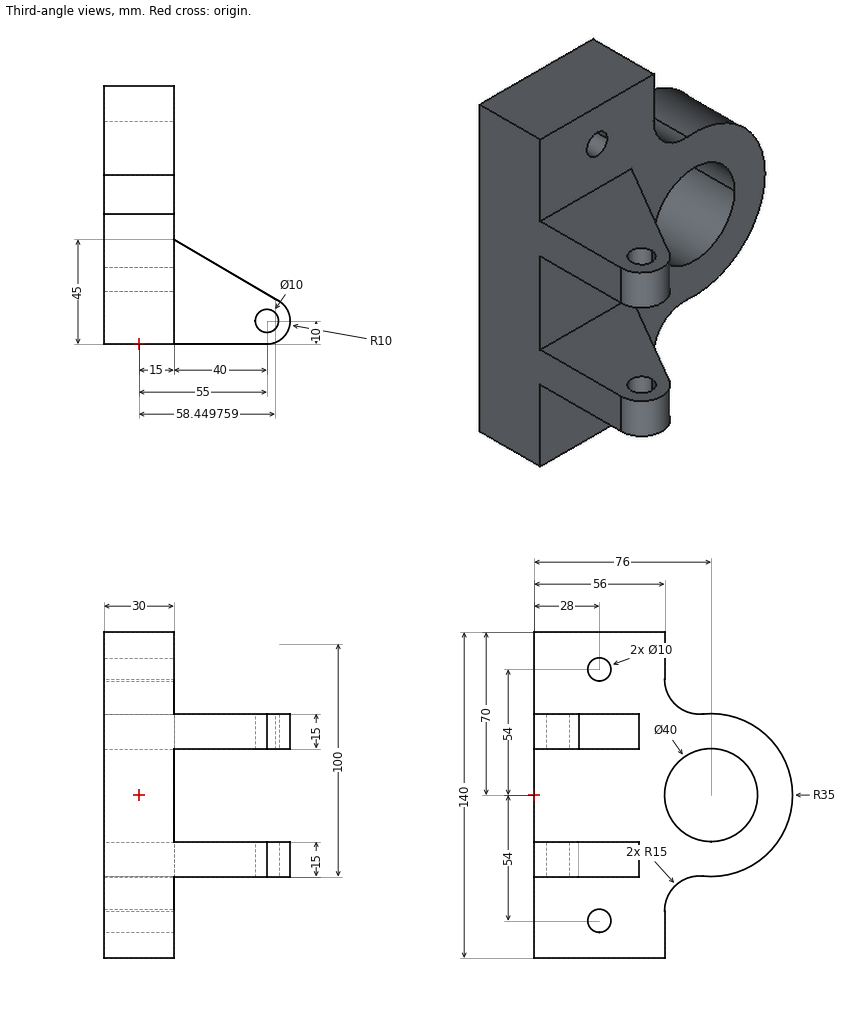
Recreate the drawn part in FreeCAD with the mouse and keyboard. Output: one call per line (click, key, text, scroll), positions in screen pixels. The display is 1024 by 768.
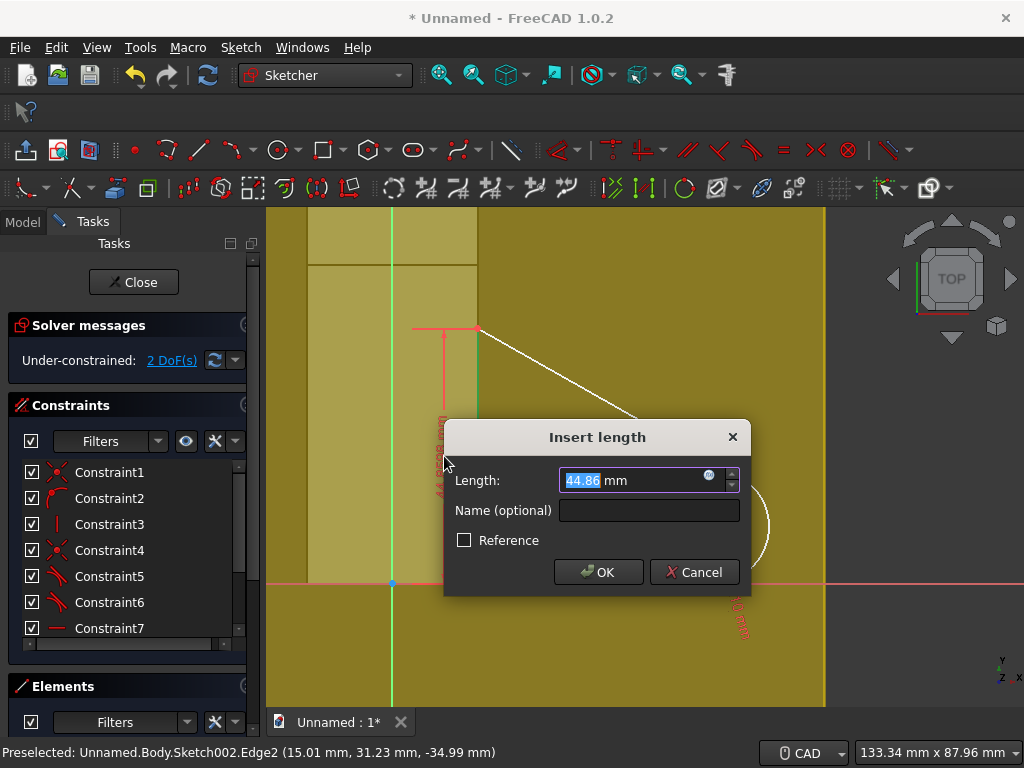
text(45)
key(Return)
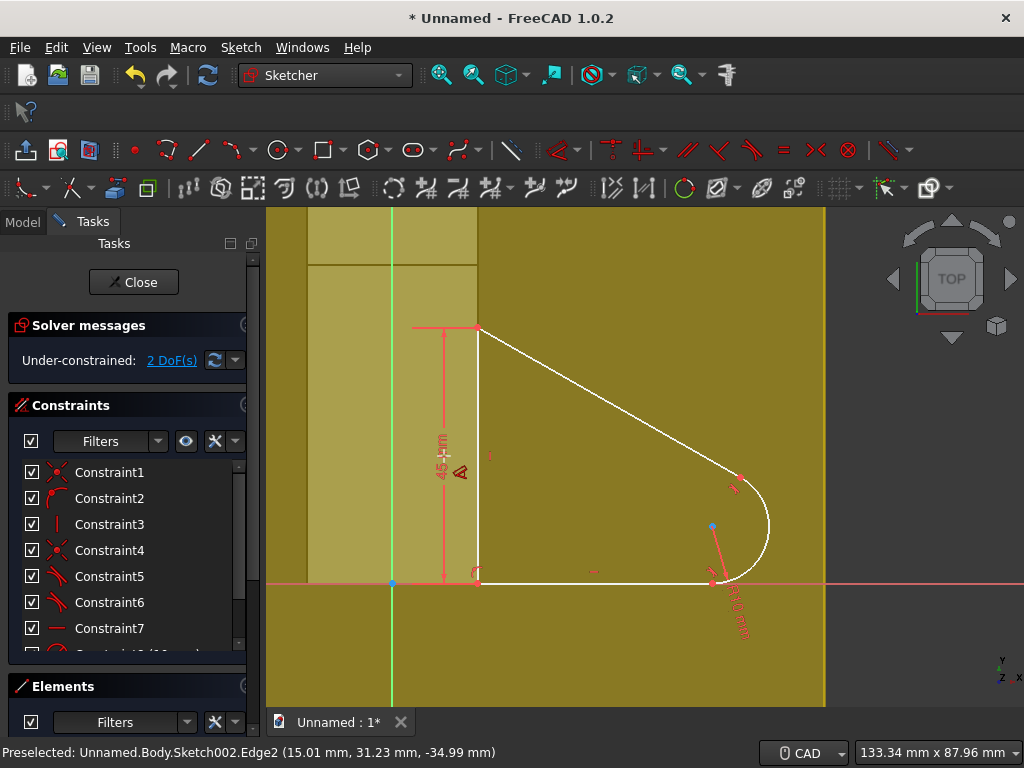
click(548, 584)
click(595, 618)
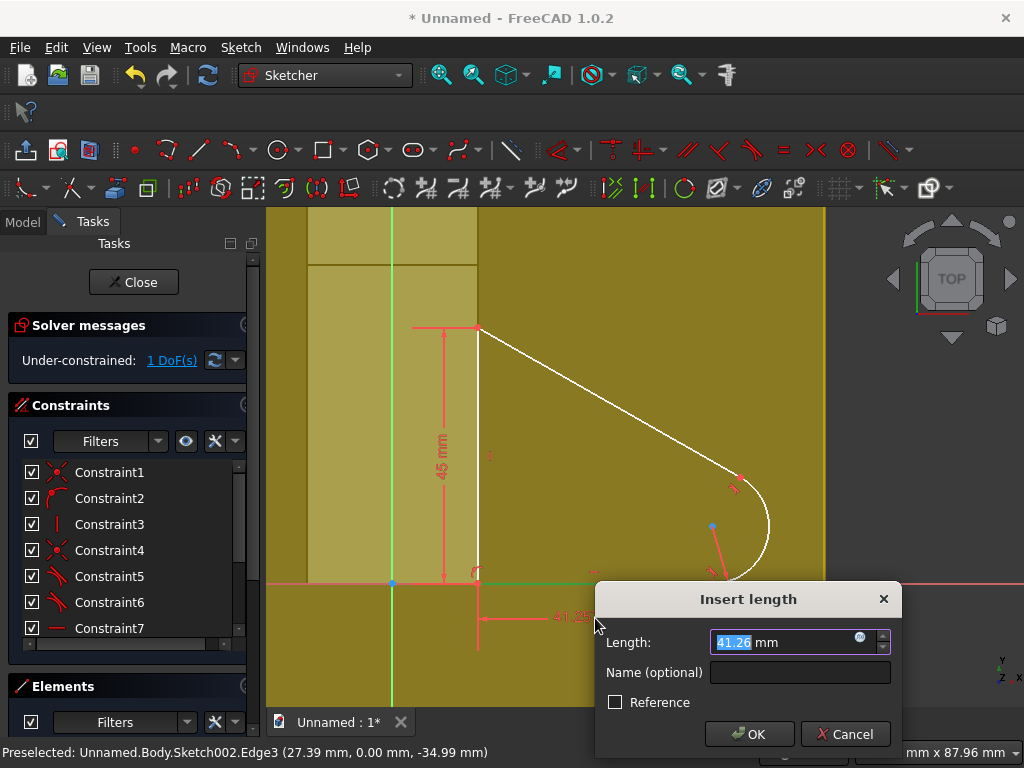
text(40)
key(Return)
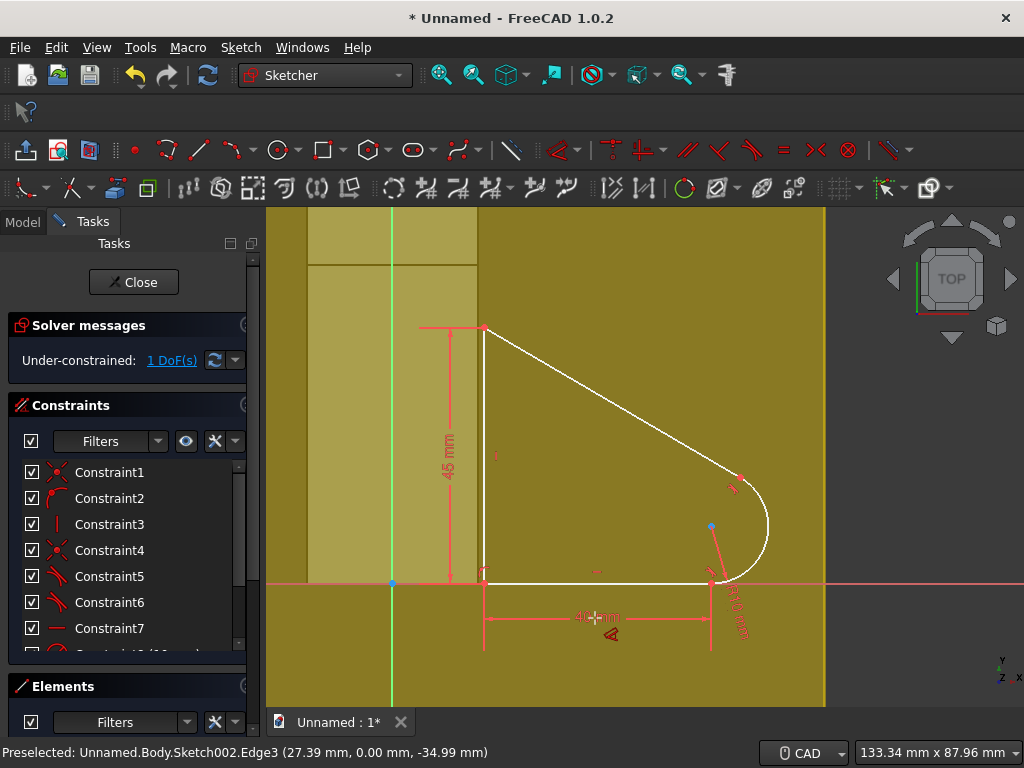
click(484, 328)
click(438, 618)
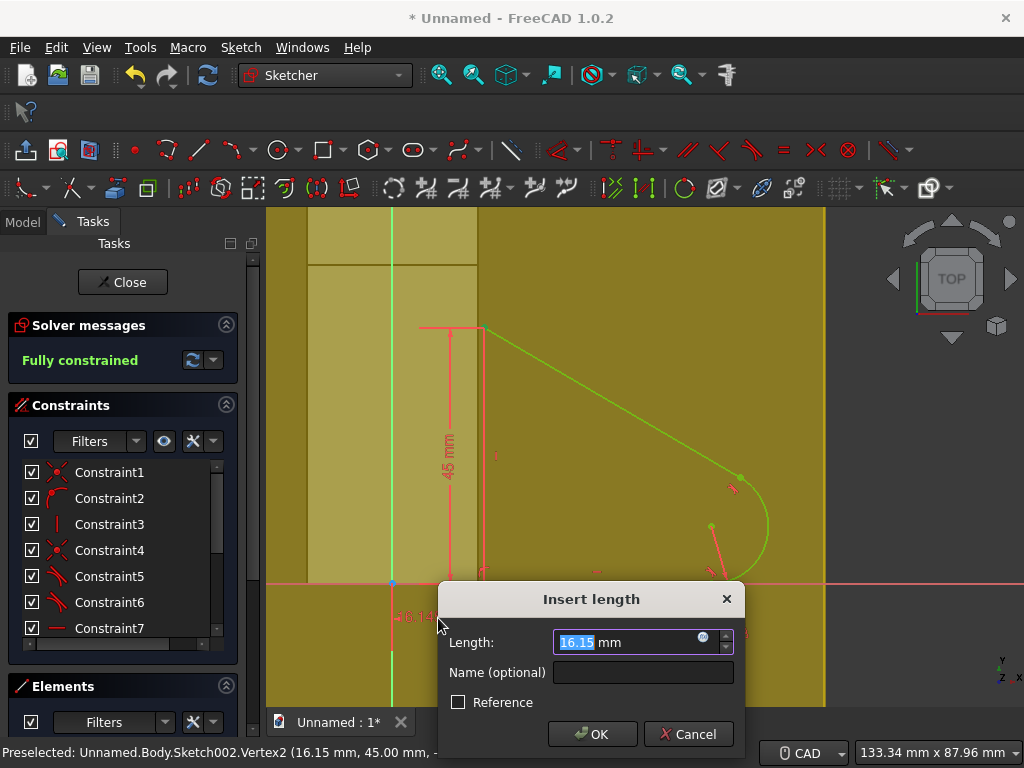
text(15)
key(Return)
key(Escape)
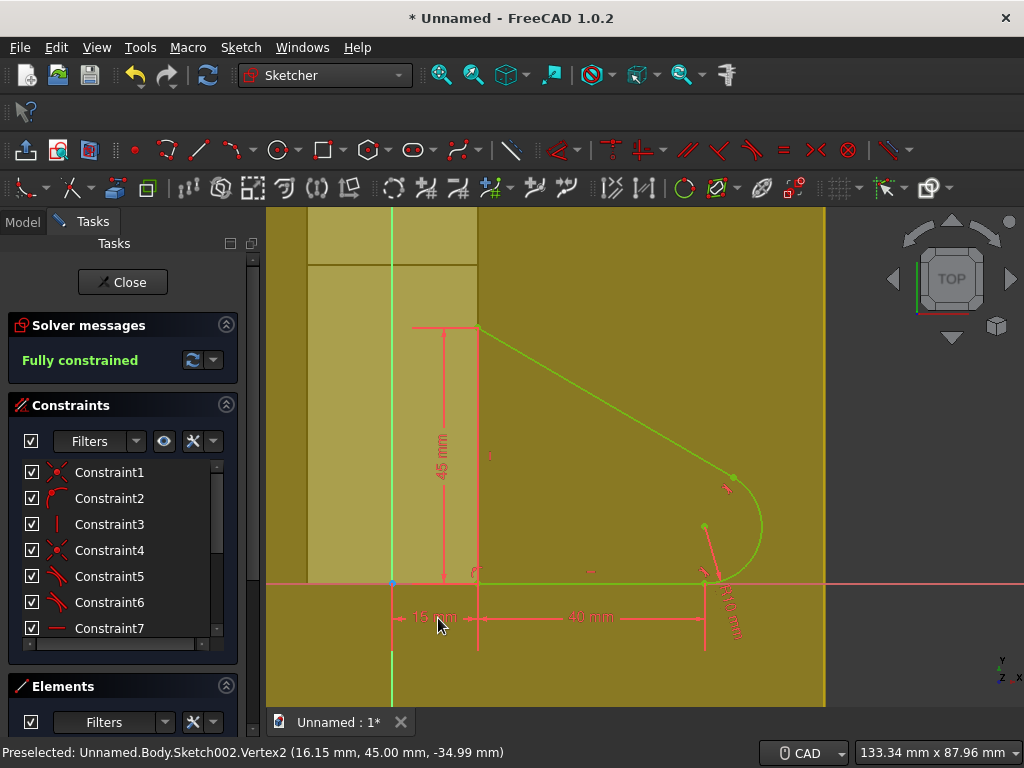
click(123, 282)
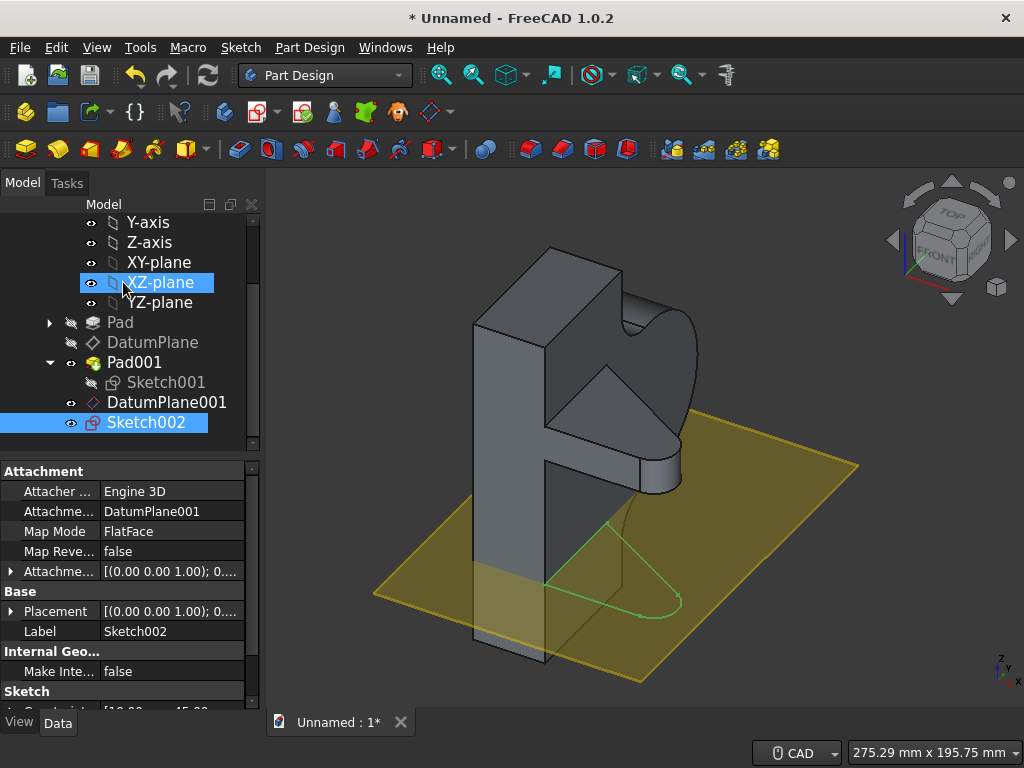
click(26, 150)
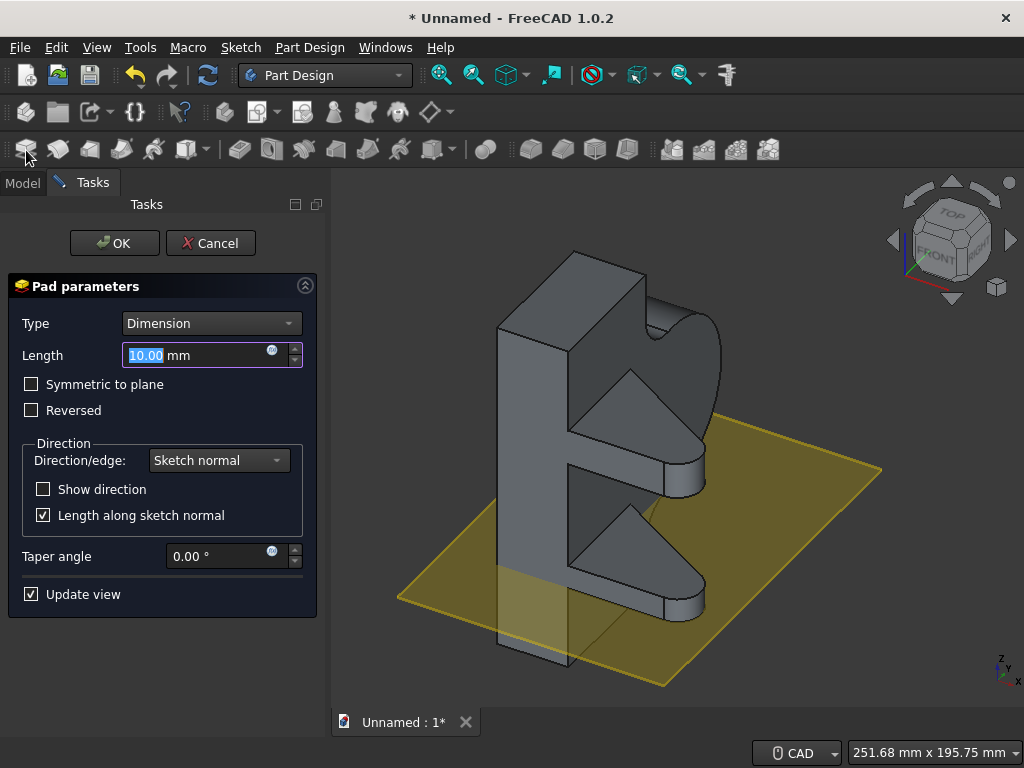
text(15)
key(Tab)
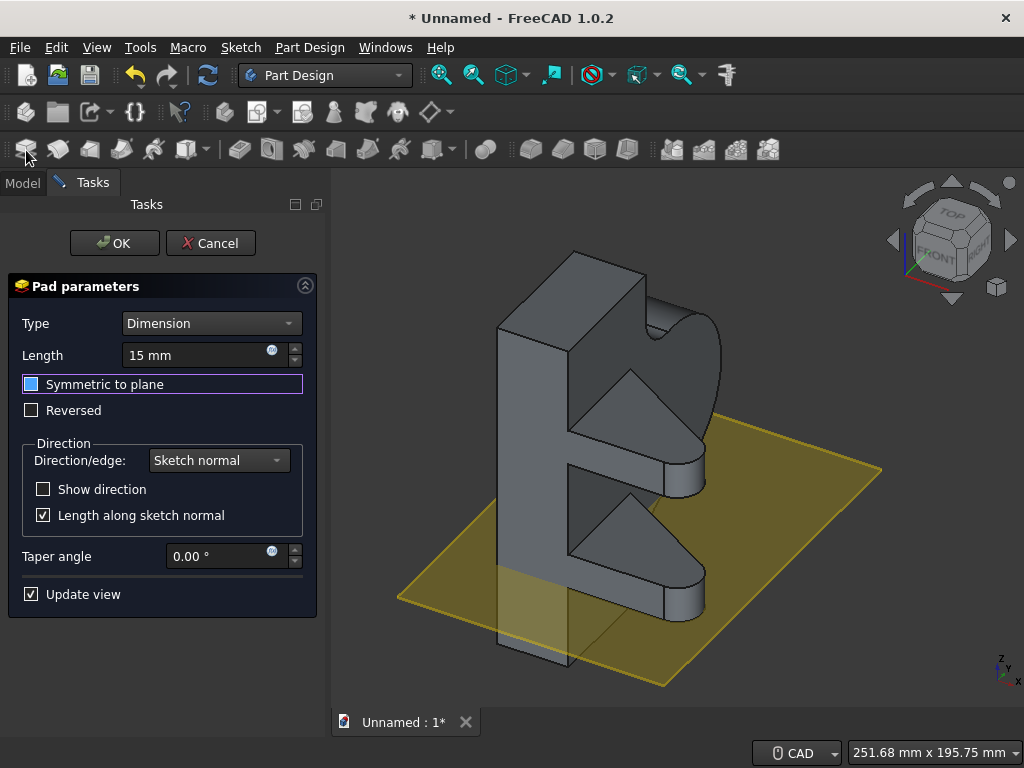
click(115, 243)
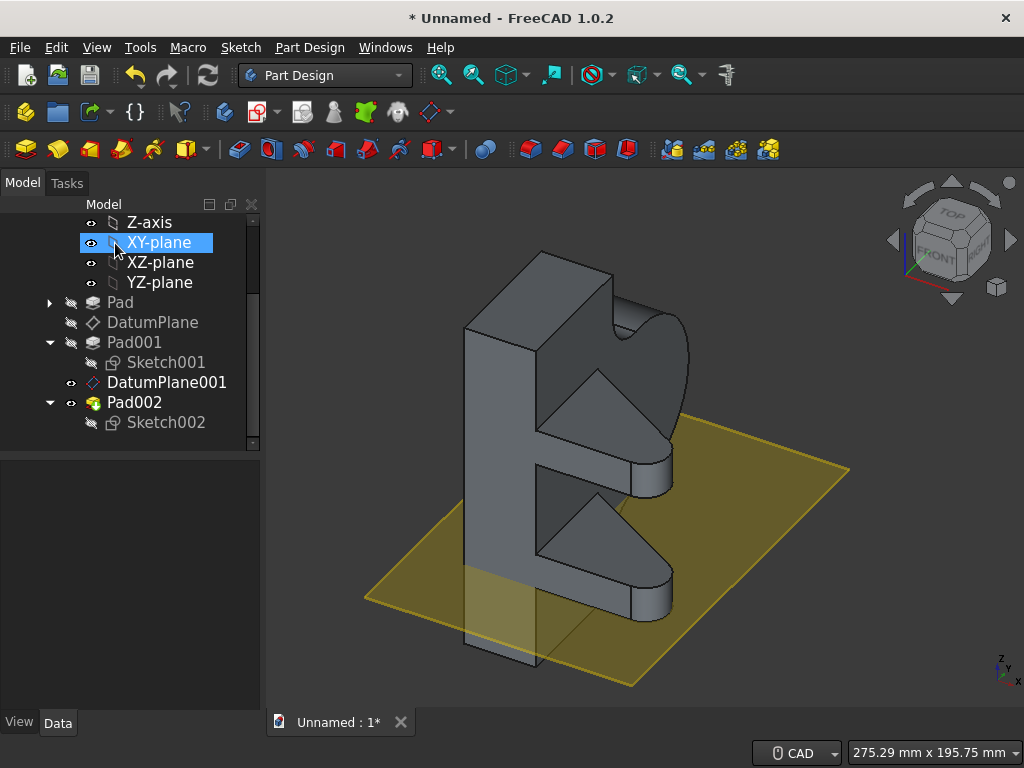
click(116, 383)
key(space)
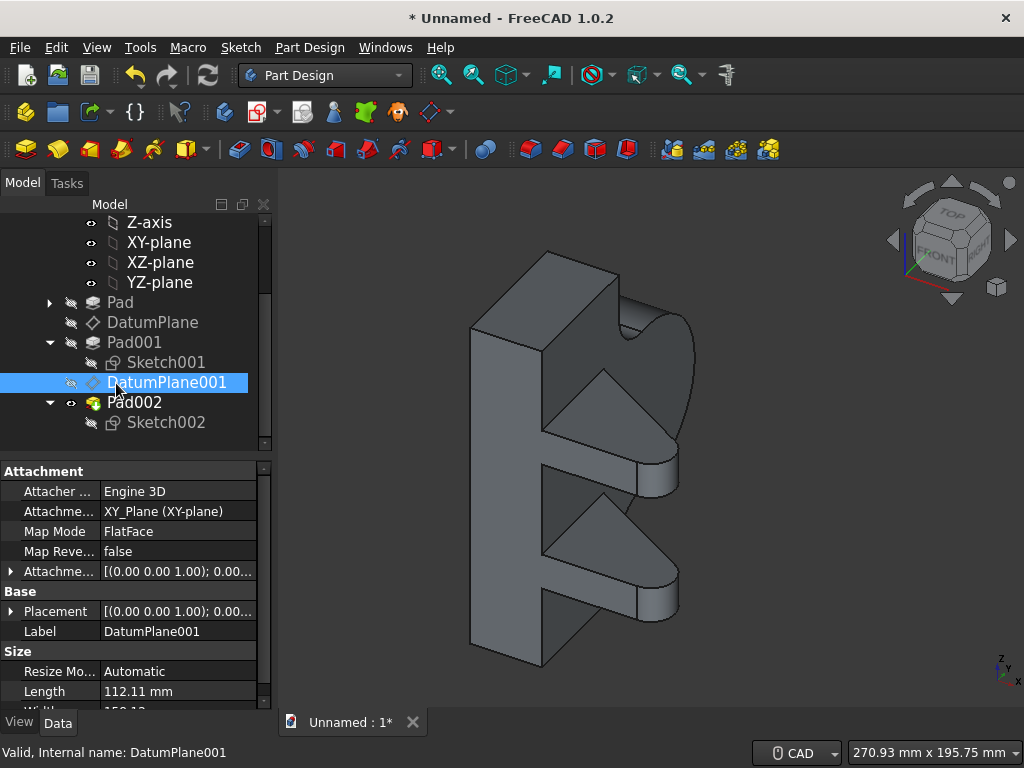
key(5)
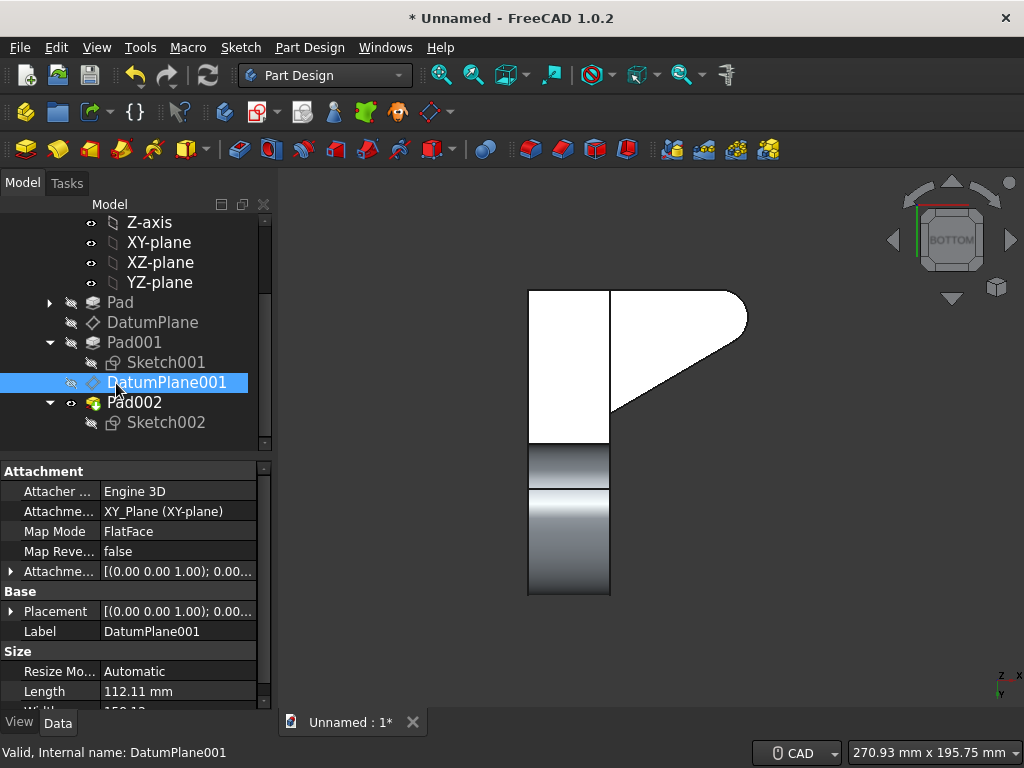
click(660, 333)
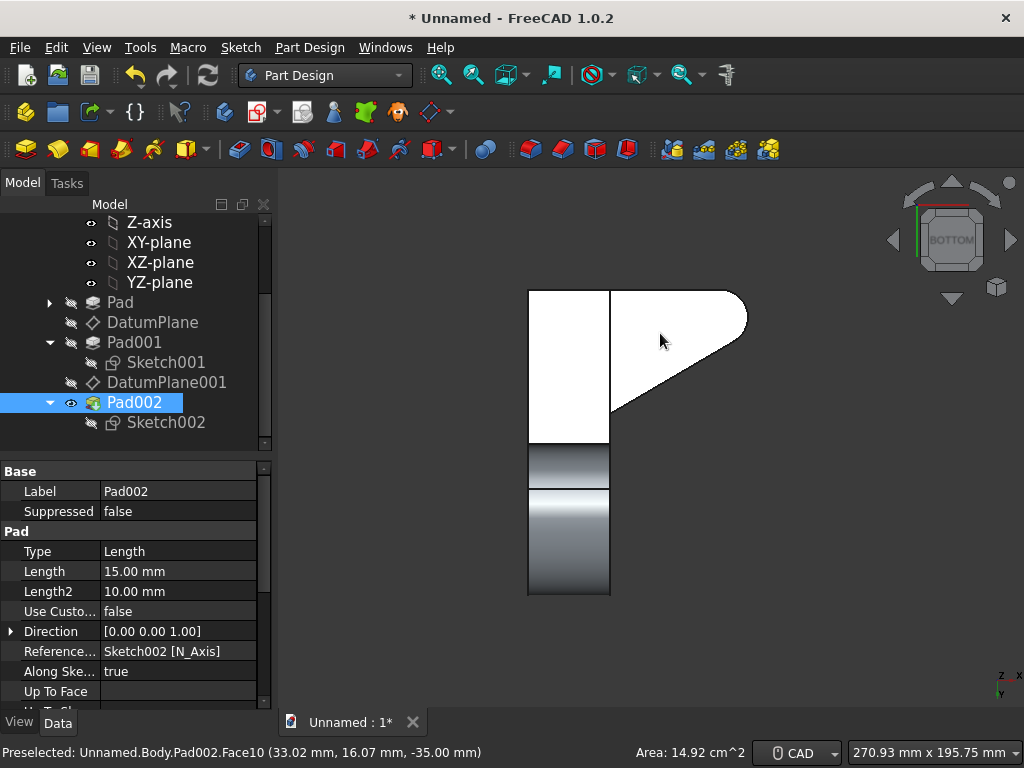
click(258, 112)